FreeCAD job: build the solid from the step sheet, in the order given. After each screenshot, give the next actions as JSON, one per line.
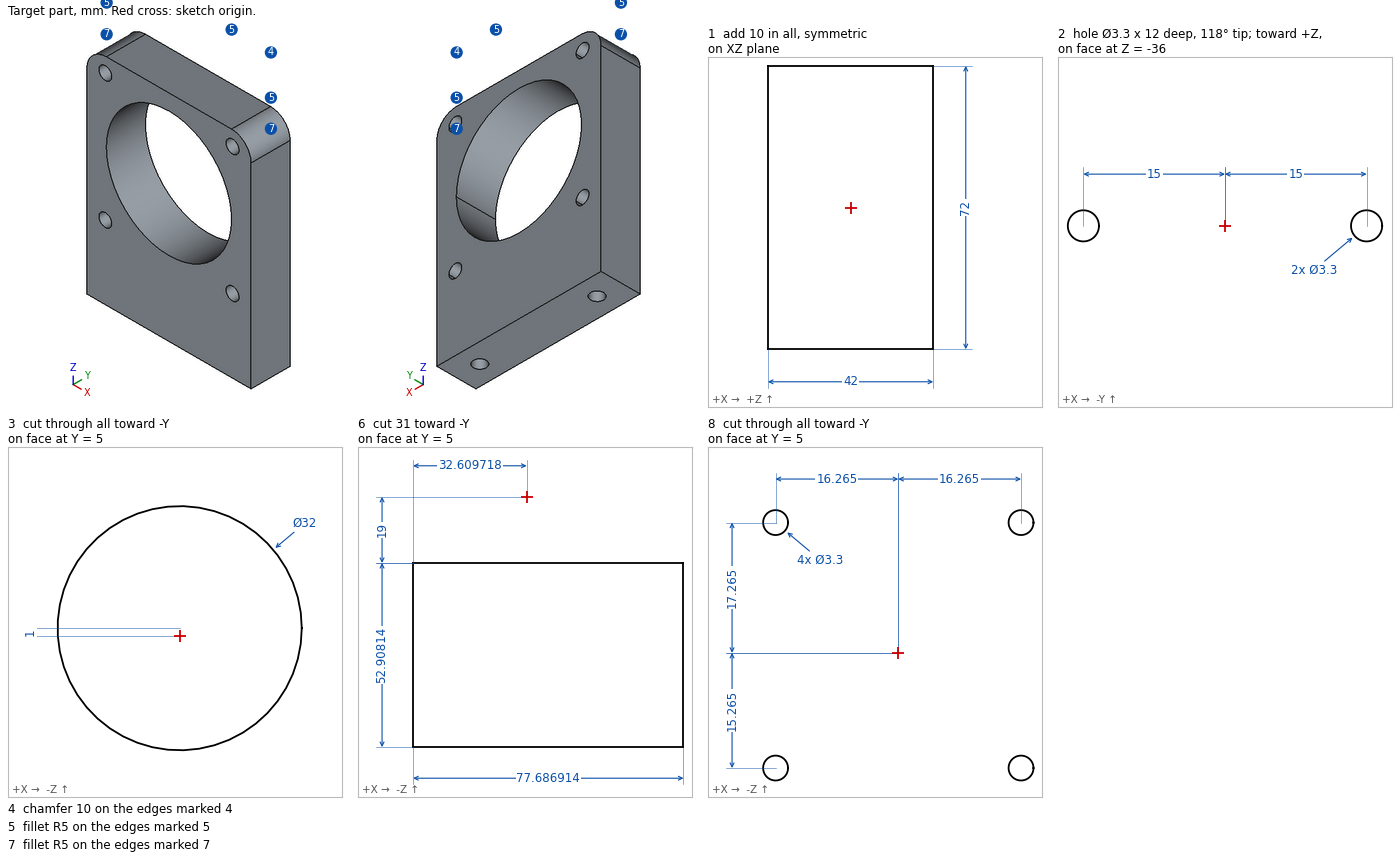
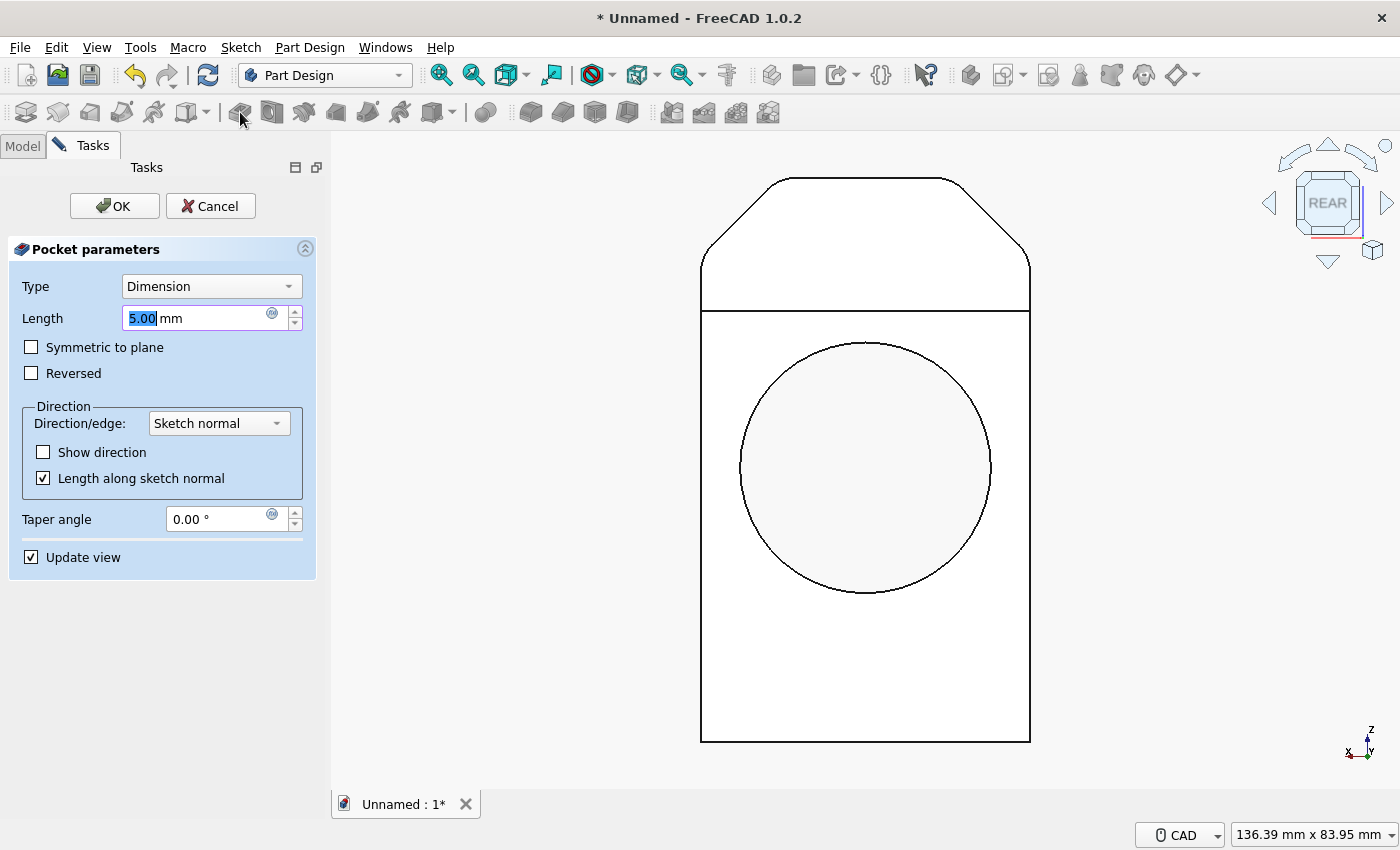
{"action": "type", "text": "31"}
{"action": "key", "text": "Tab"}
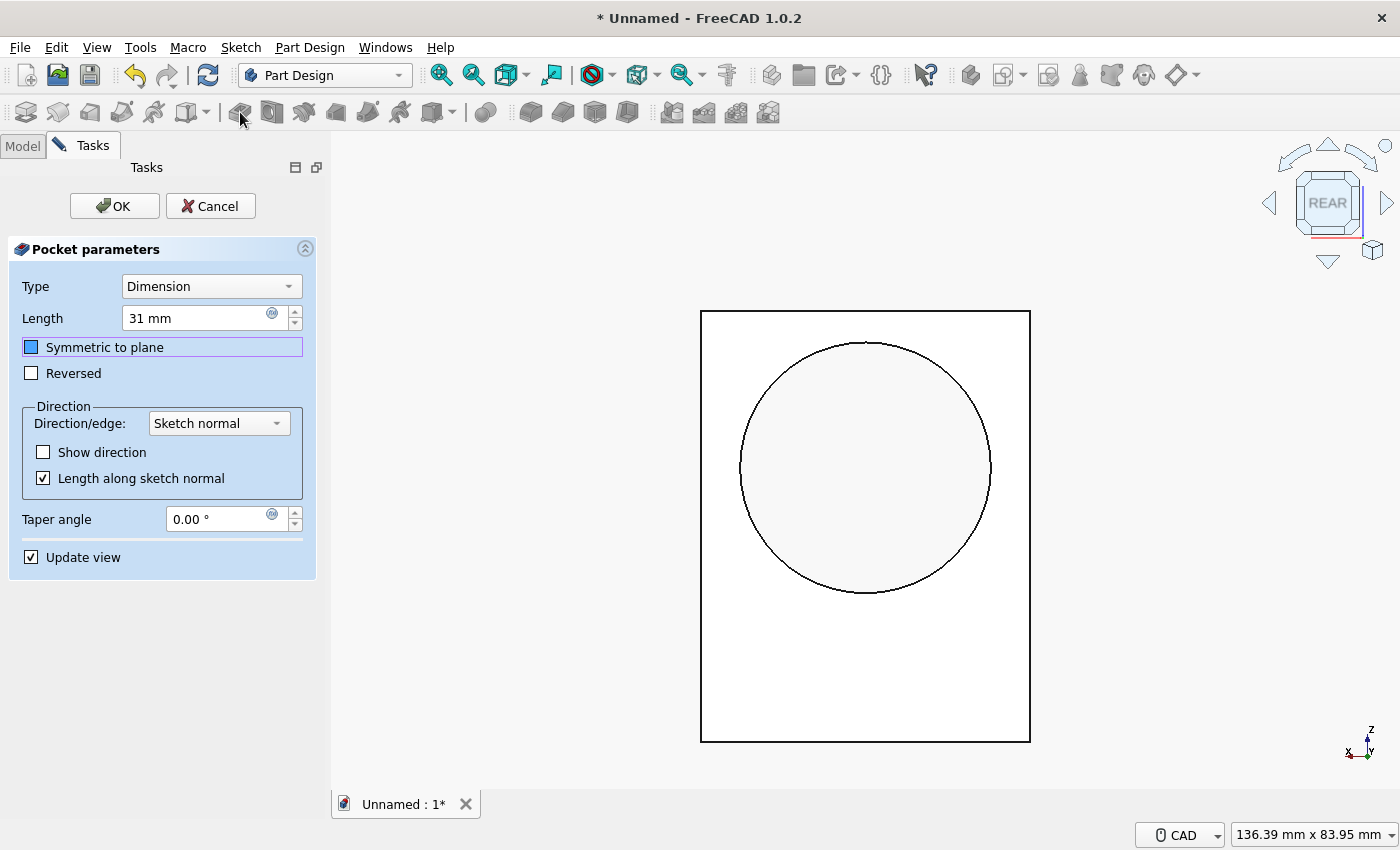
{"action": "left_click", "coordinate": [115, 206]}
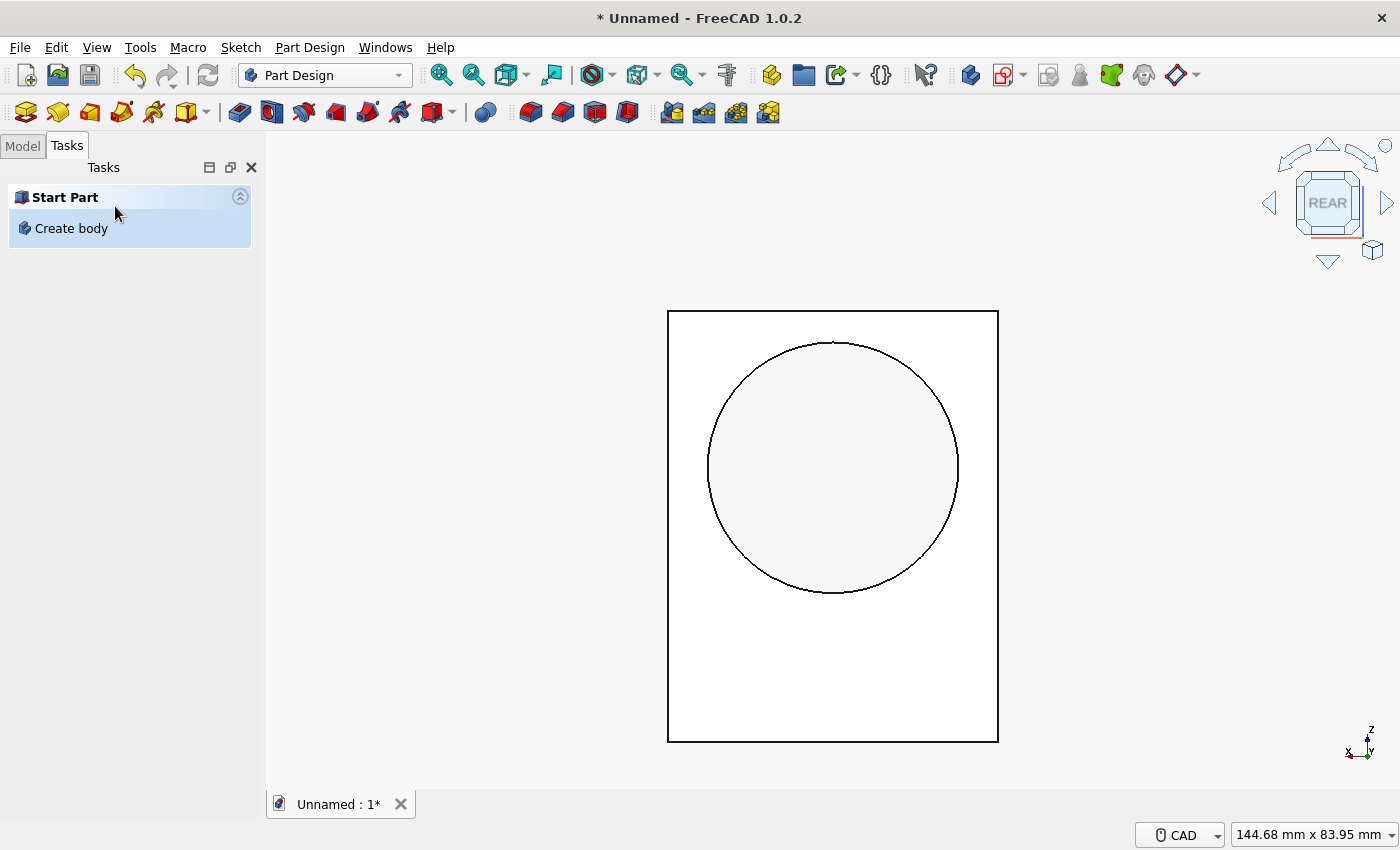
{"action": "key", "text": "0"}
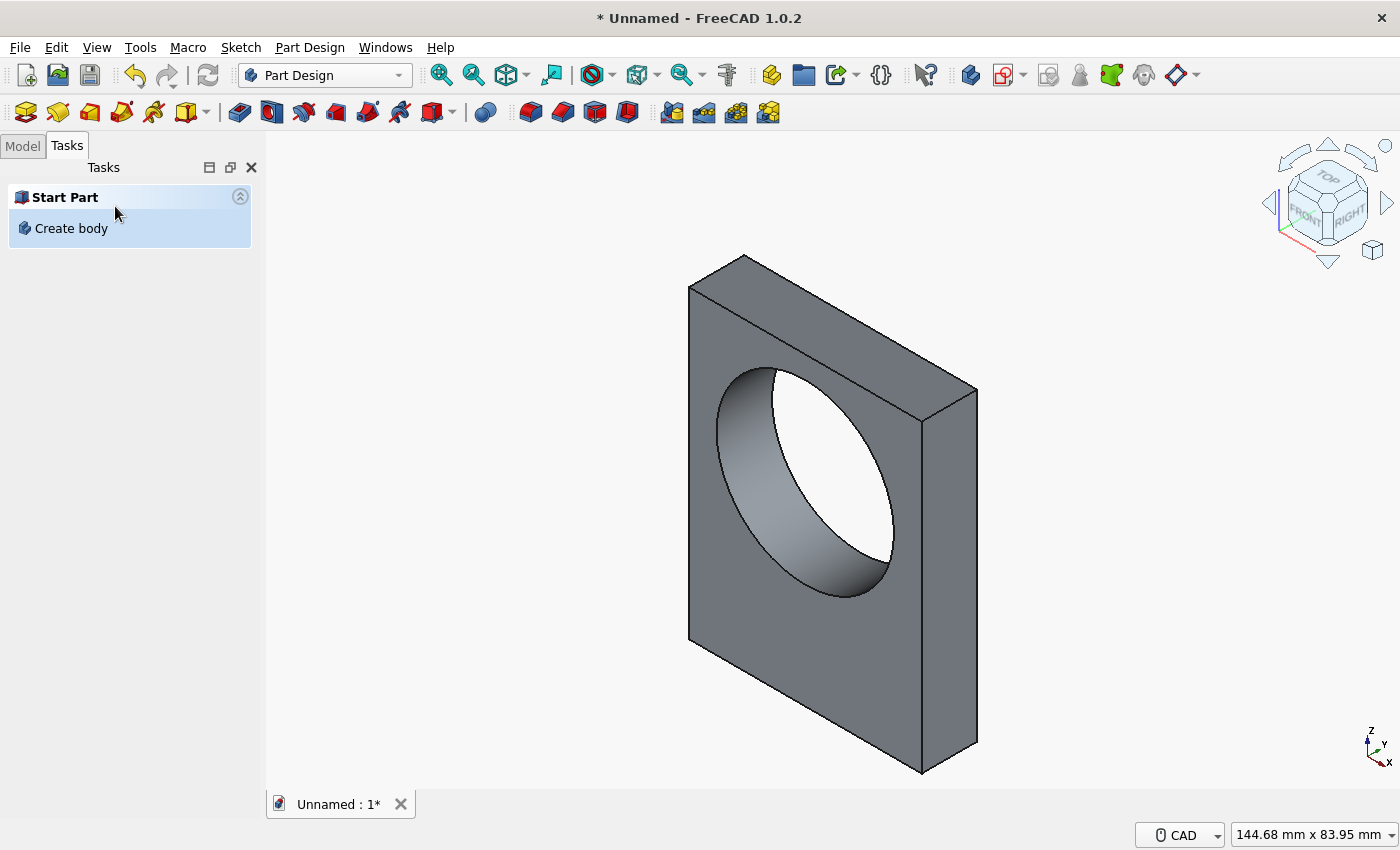
{"action": "left_click", "coordinate": [949, 405]}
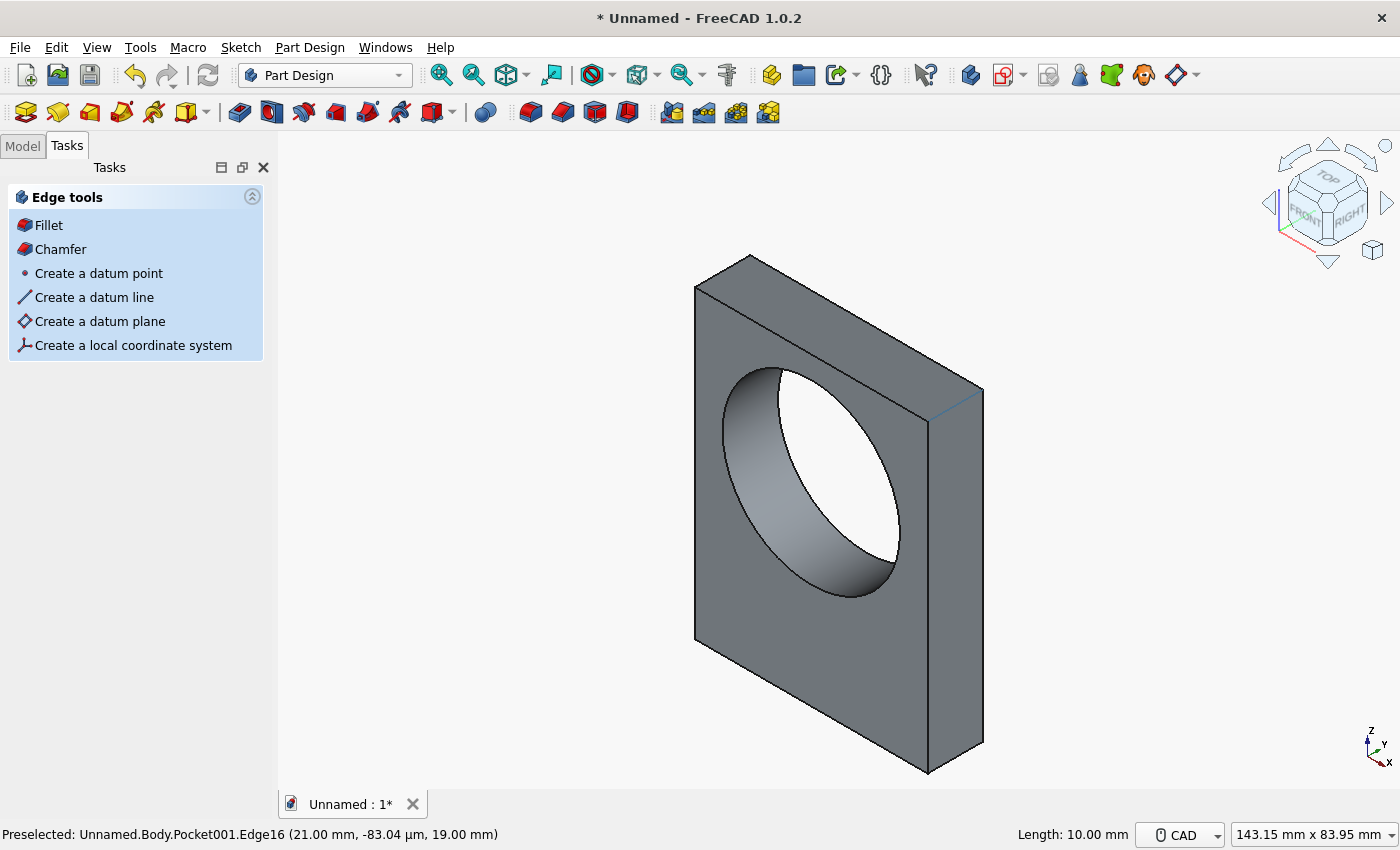
{"action": "key", "text": "2"}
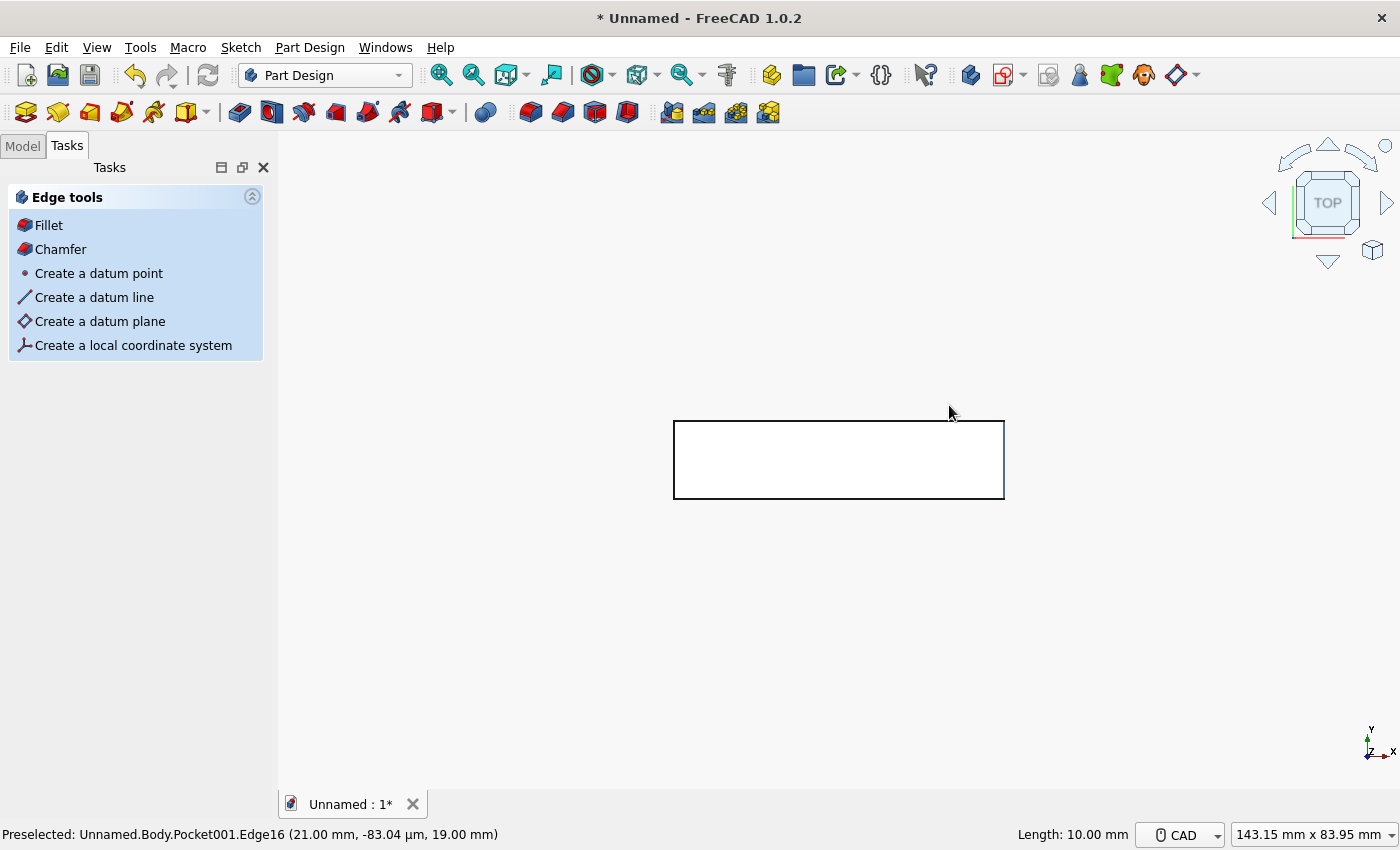
{"action": "left_click", "coordinate": [442, 76]}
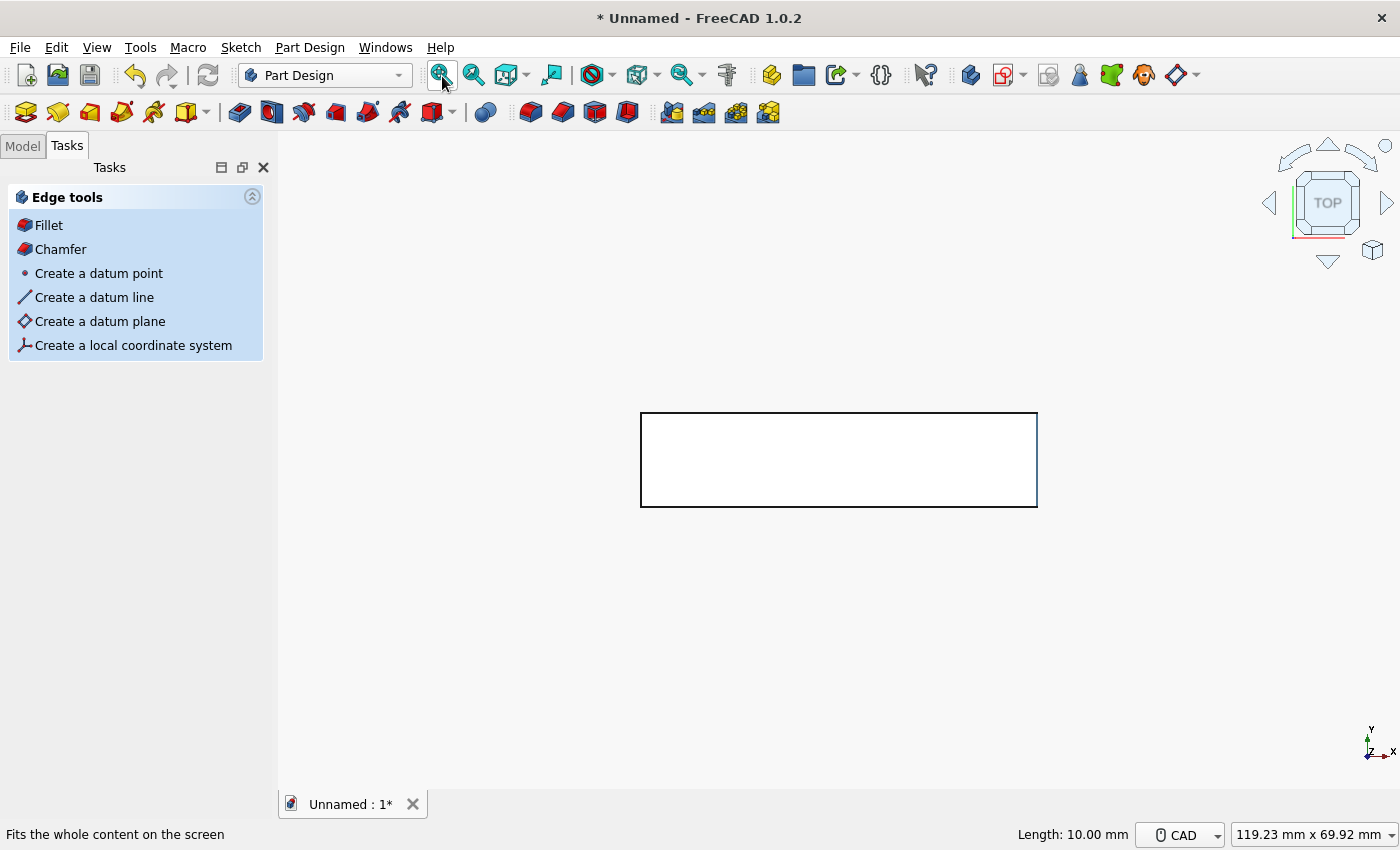
{"action": "left_click", "coordinate": [641, 459], "text": "ctrl"}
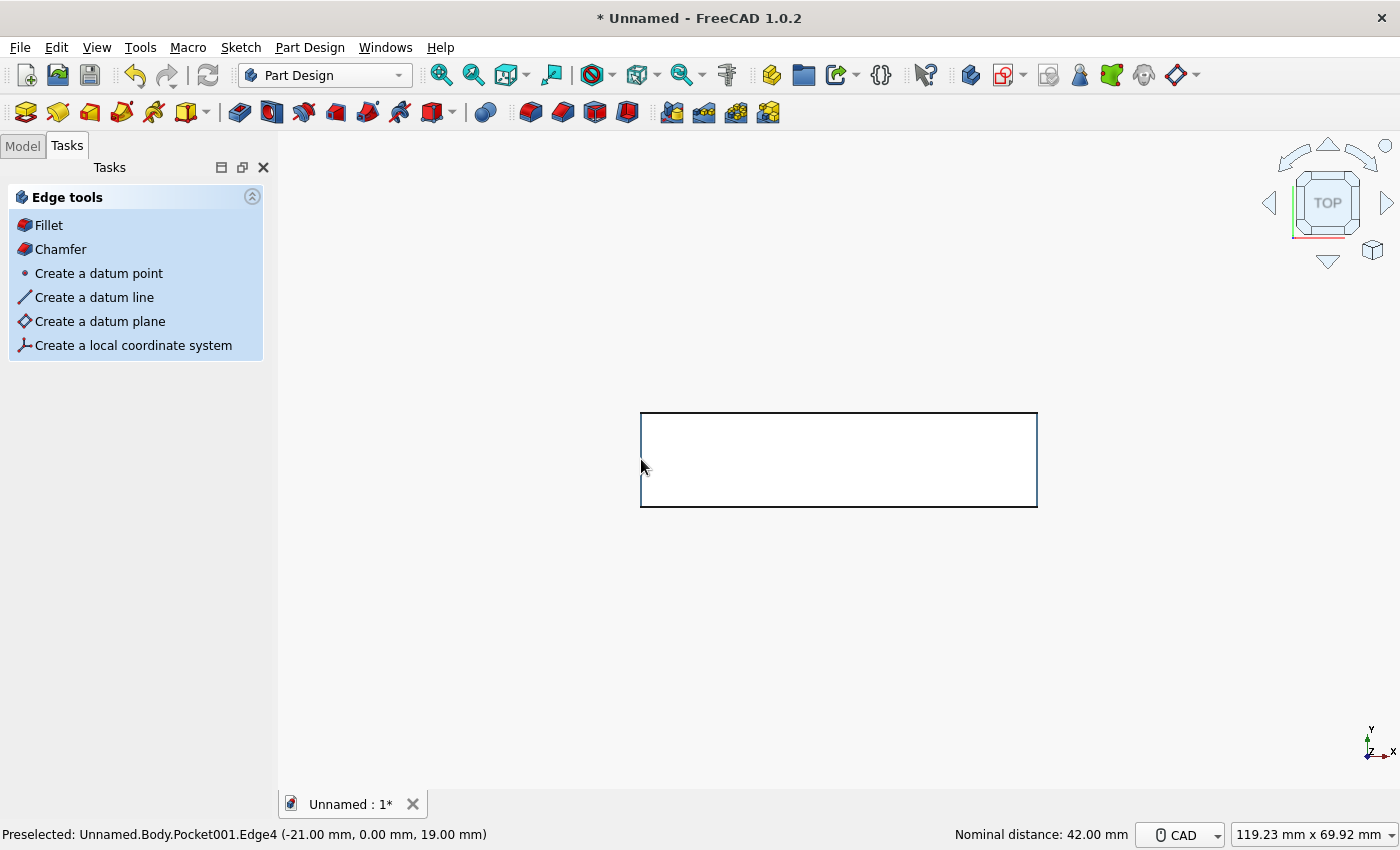
{"action": "left_click", "coordinate": [532, 112]}